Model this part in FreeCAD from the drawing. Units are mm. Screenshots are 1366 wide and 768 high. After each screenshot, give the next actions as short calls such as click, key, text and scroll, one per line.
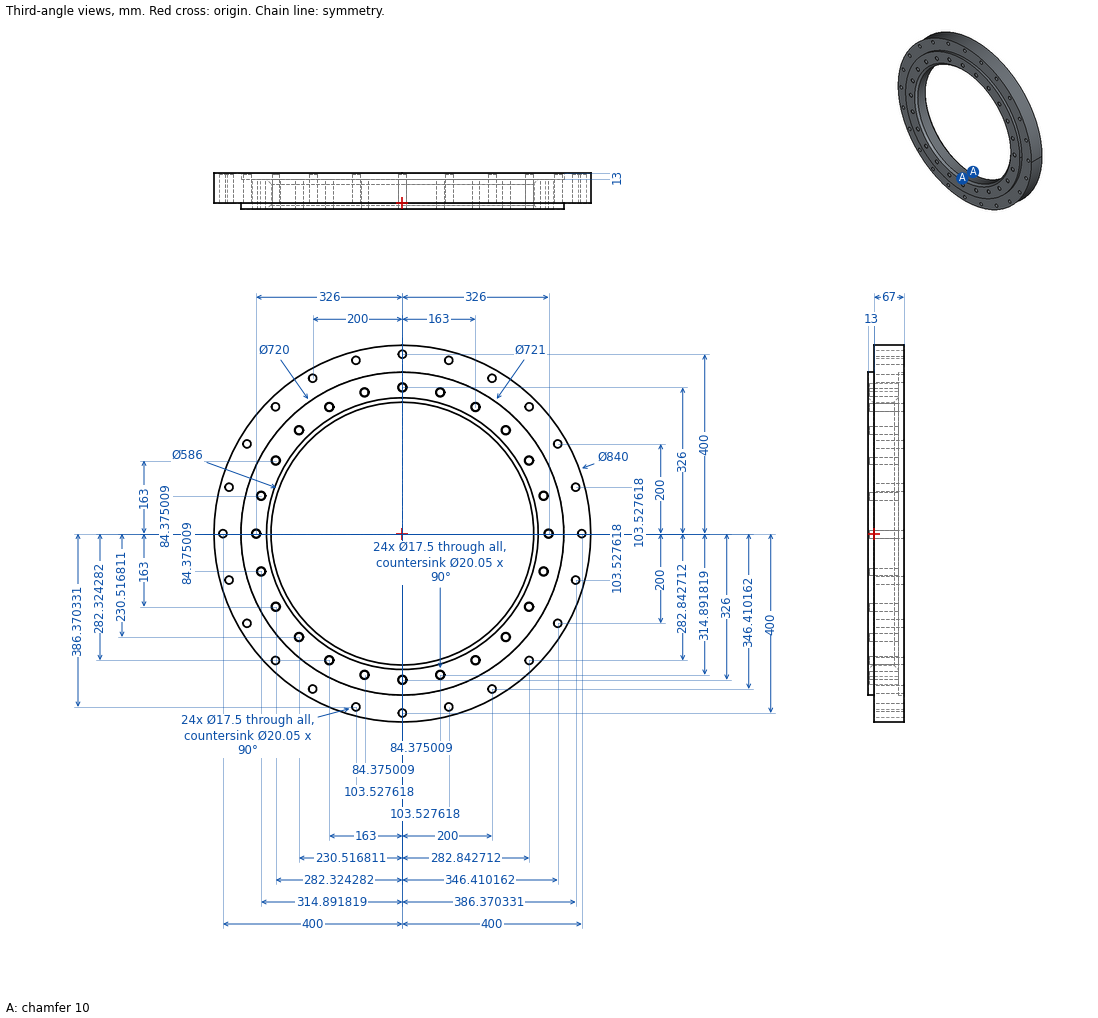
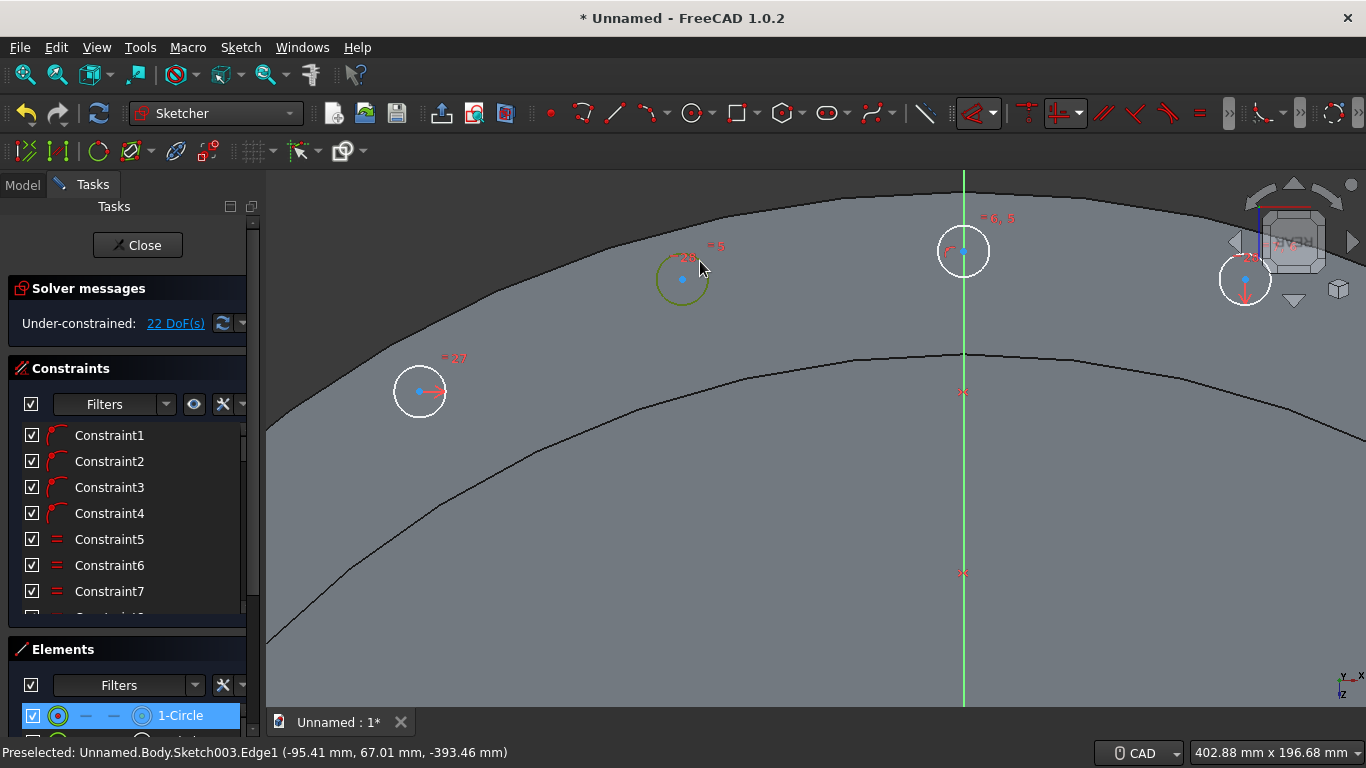
click(996, 114)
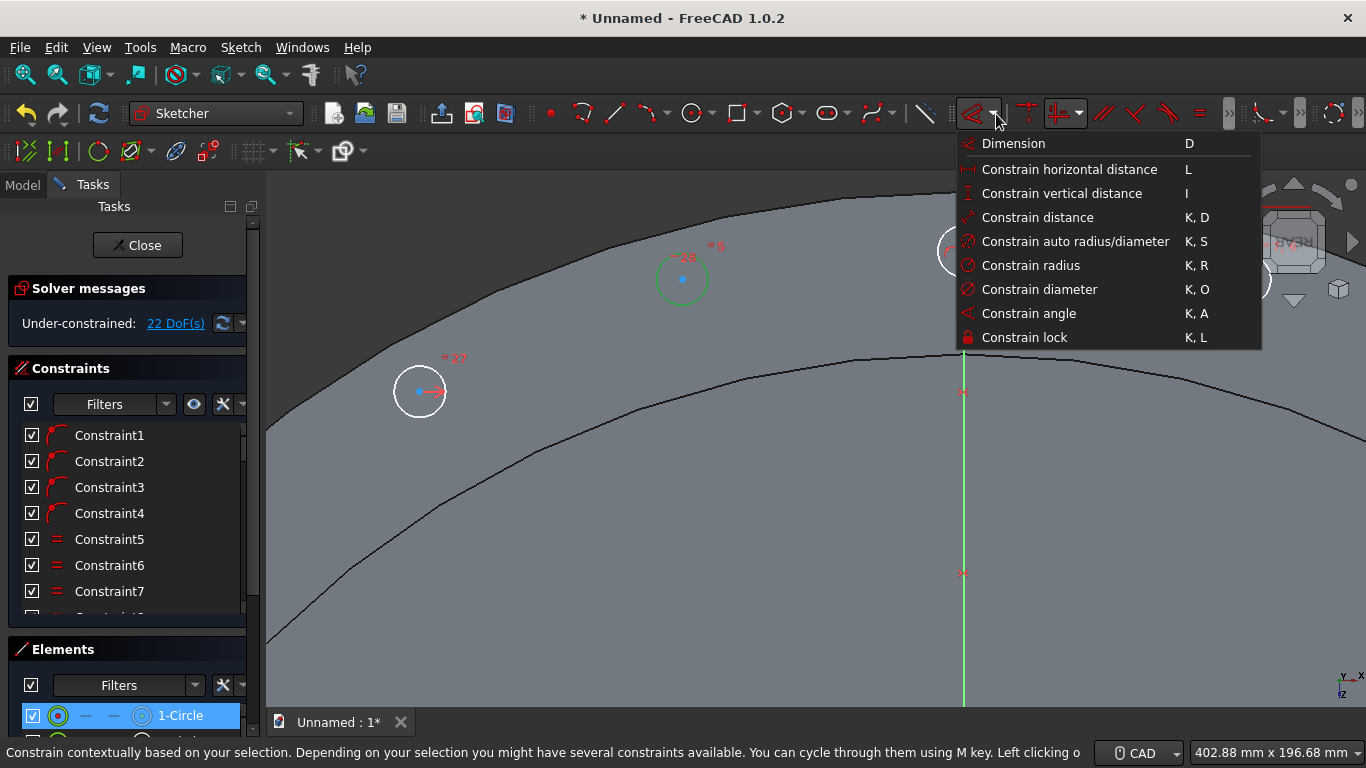
click(1109, 289)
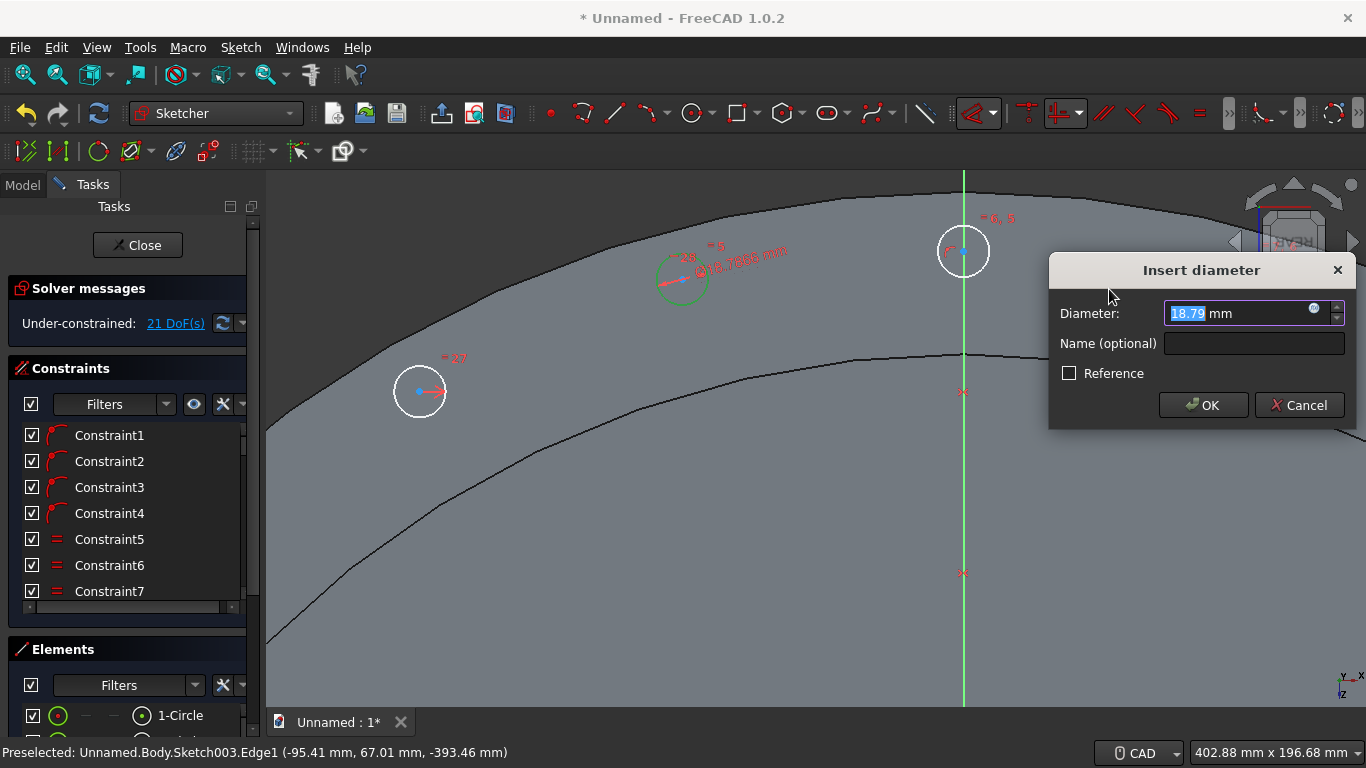
text(17.5)
key(Return)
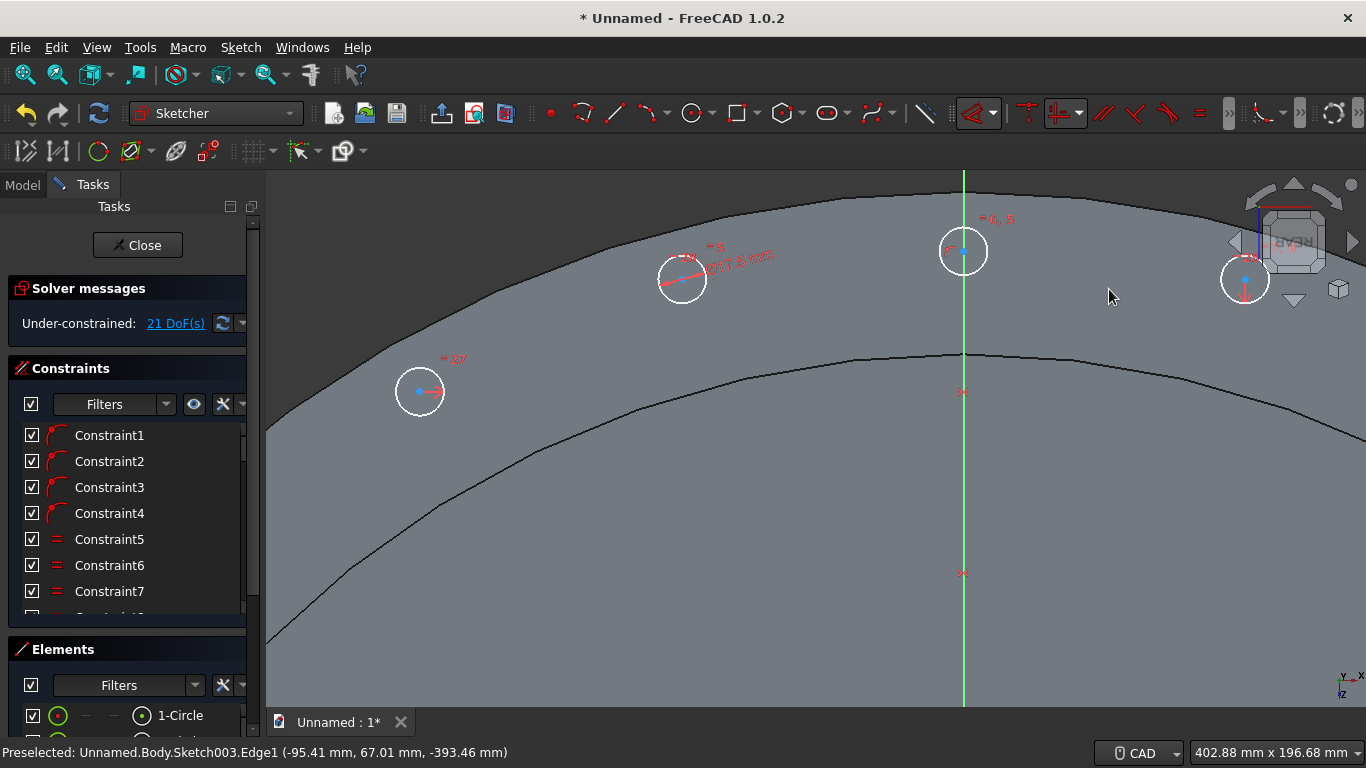
scroll(705, 260, down, 9)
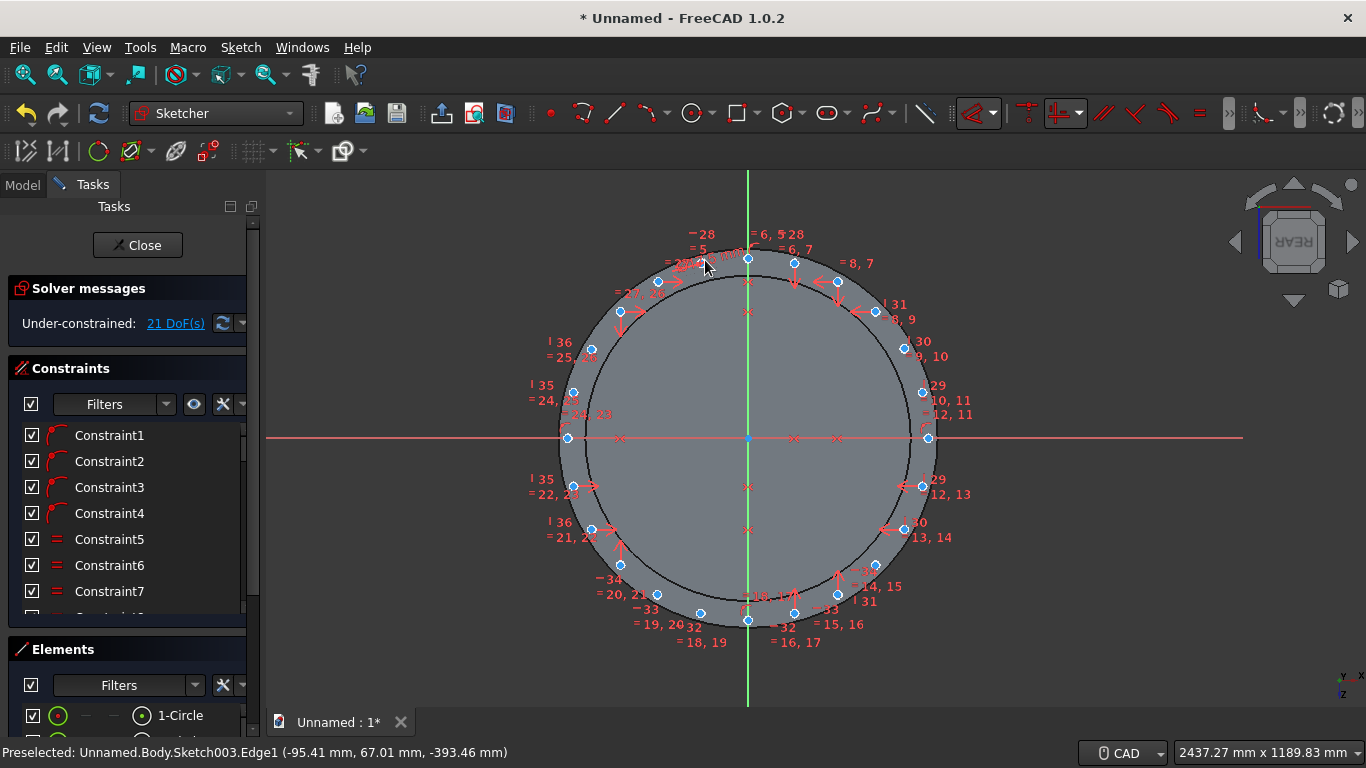
click(748, 259)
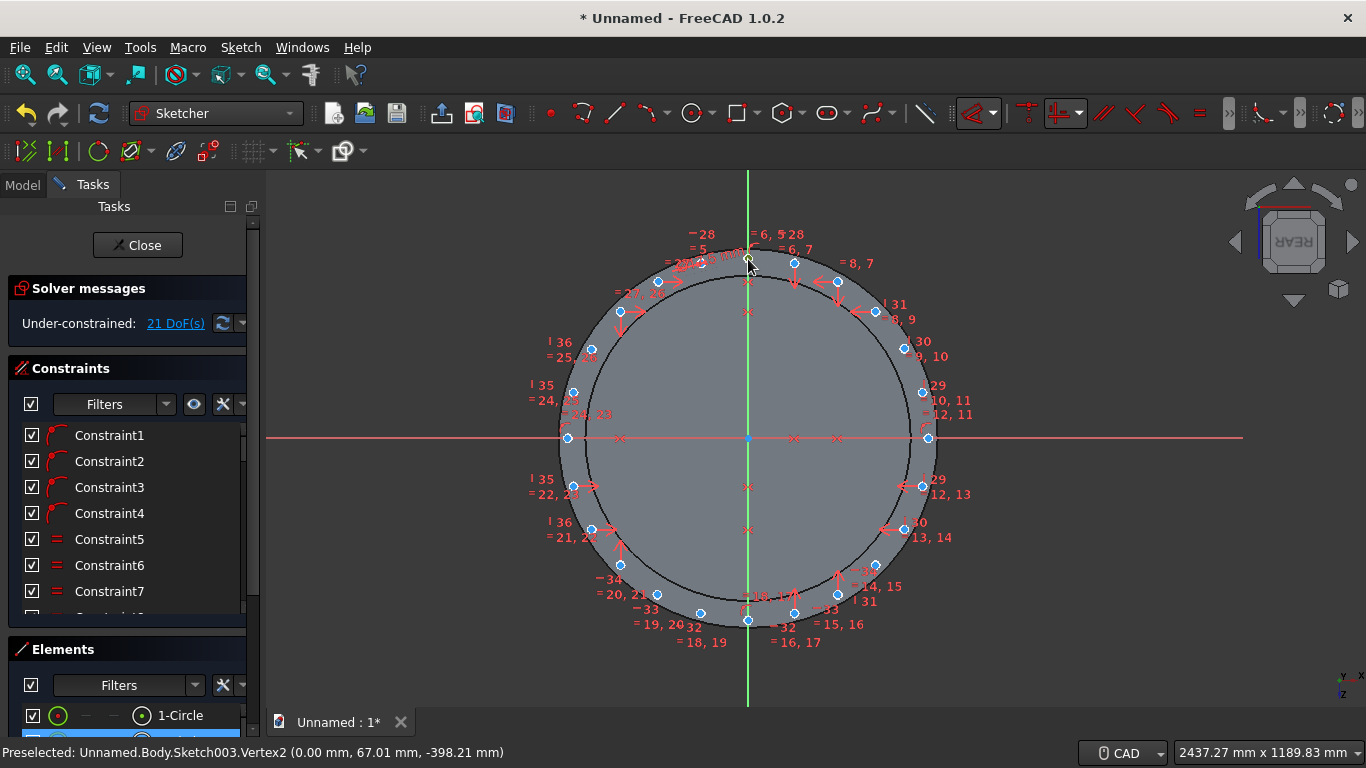
key(i)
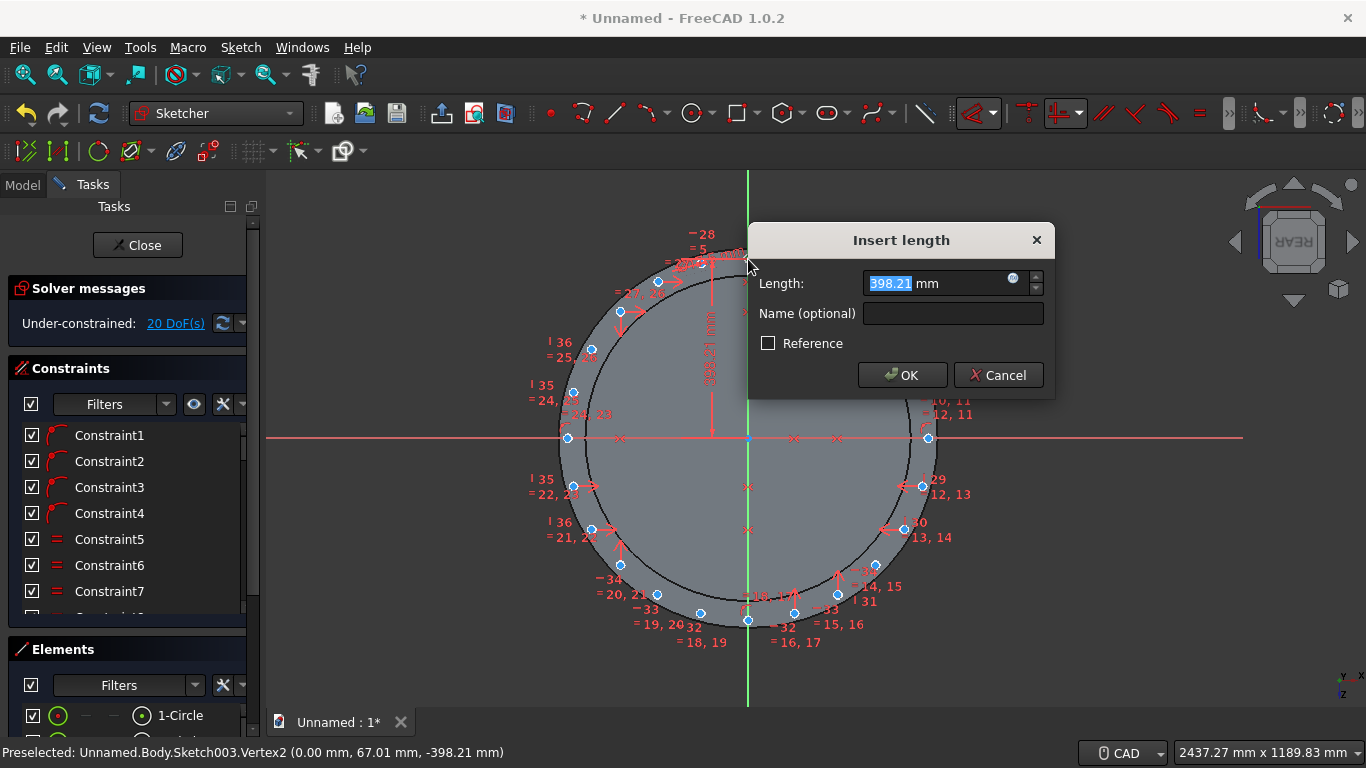
text(400)
key(Return)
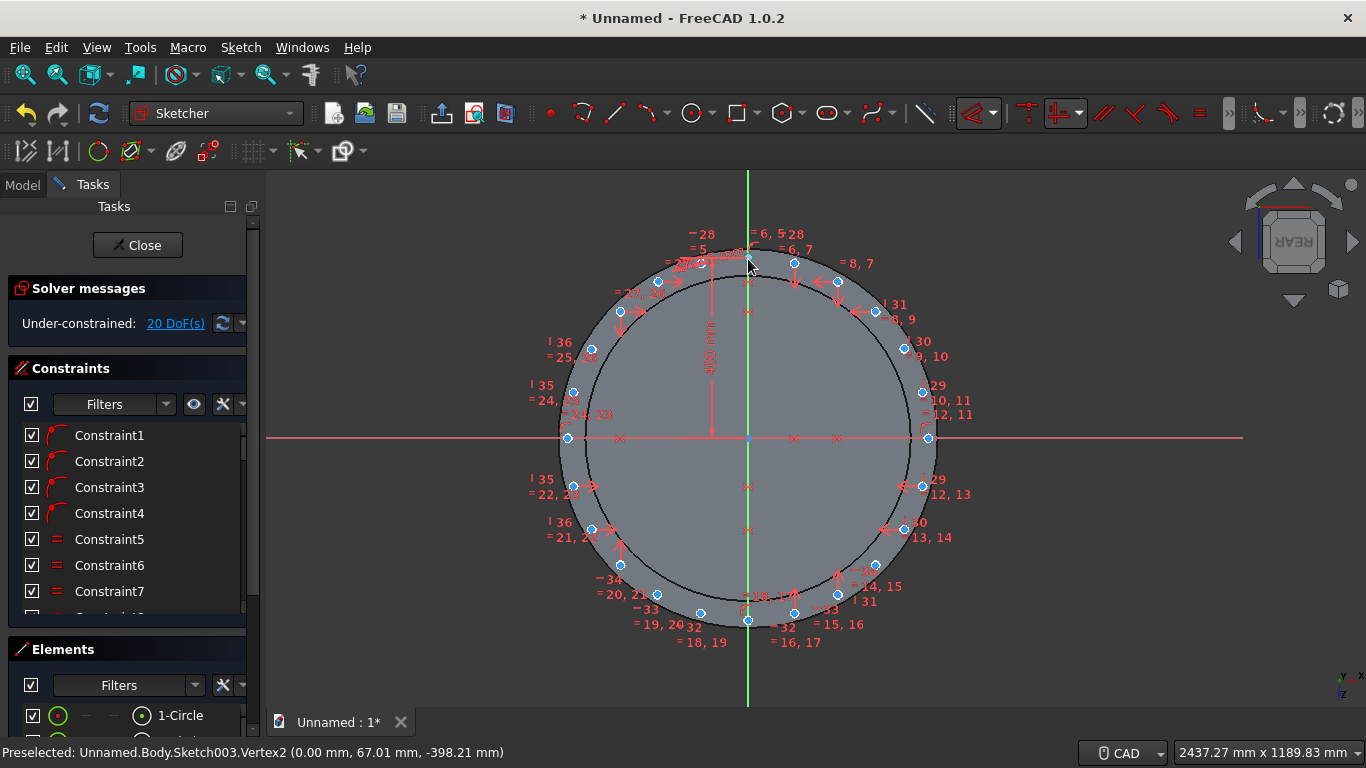
click(838, 282)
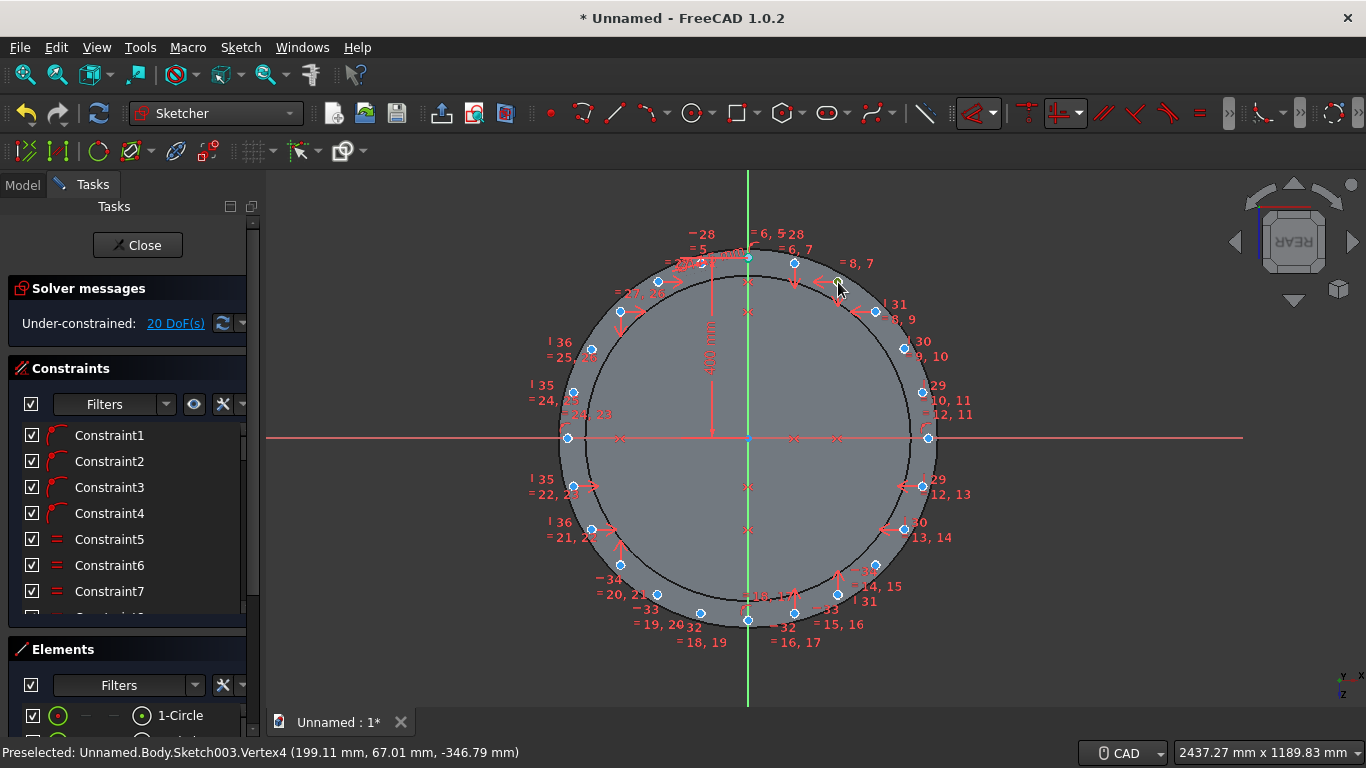
key(l)